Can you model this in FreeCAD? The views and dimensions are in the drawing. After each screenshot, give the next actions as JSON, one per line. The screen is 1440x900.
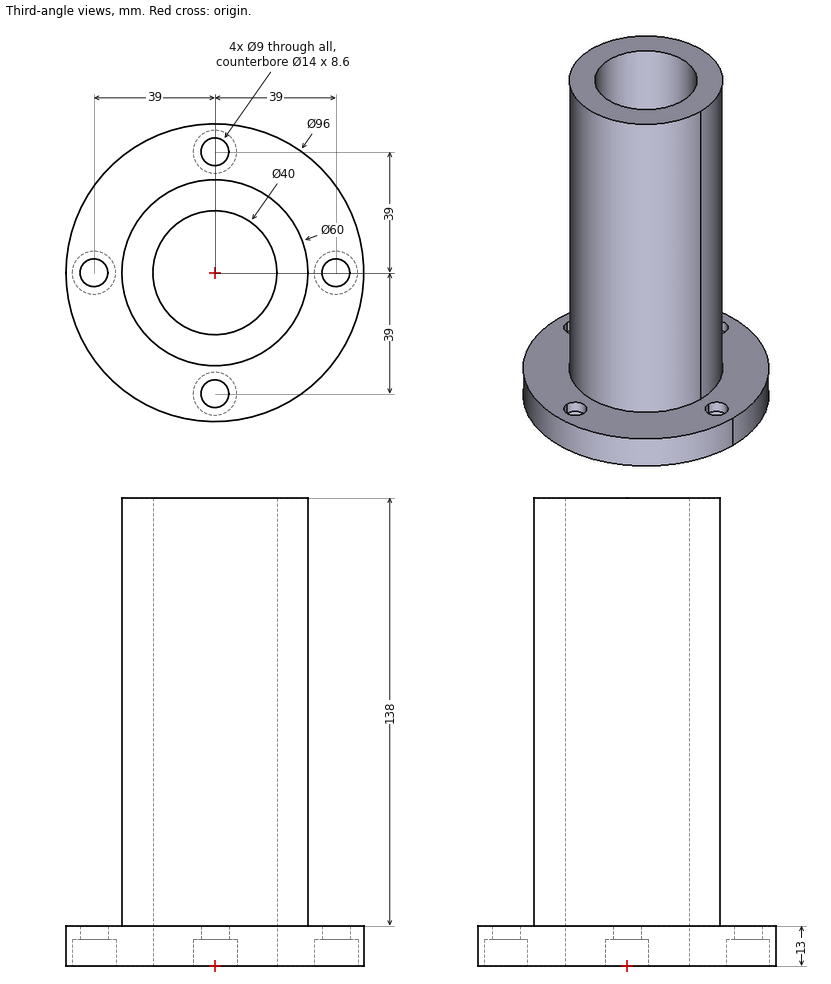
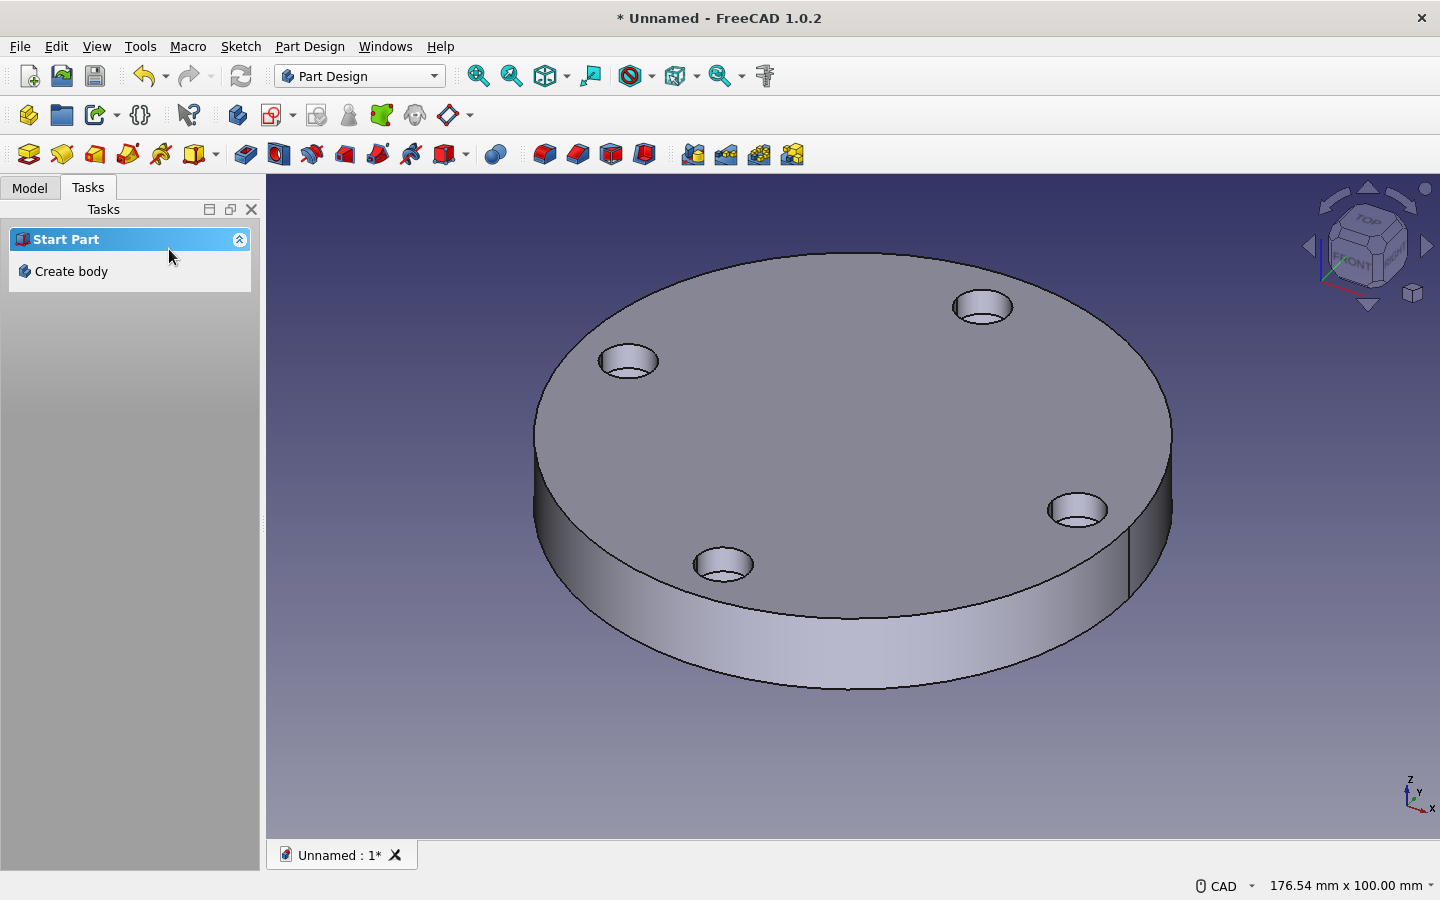
{"action": "left_click", "coordinate": [853, 435]}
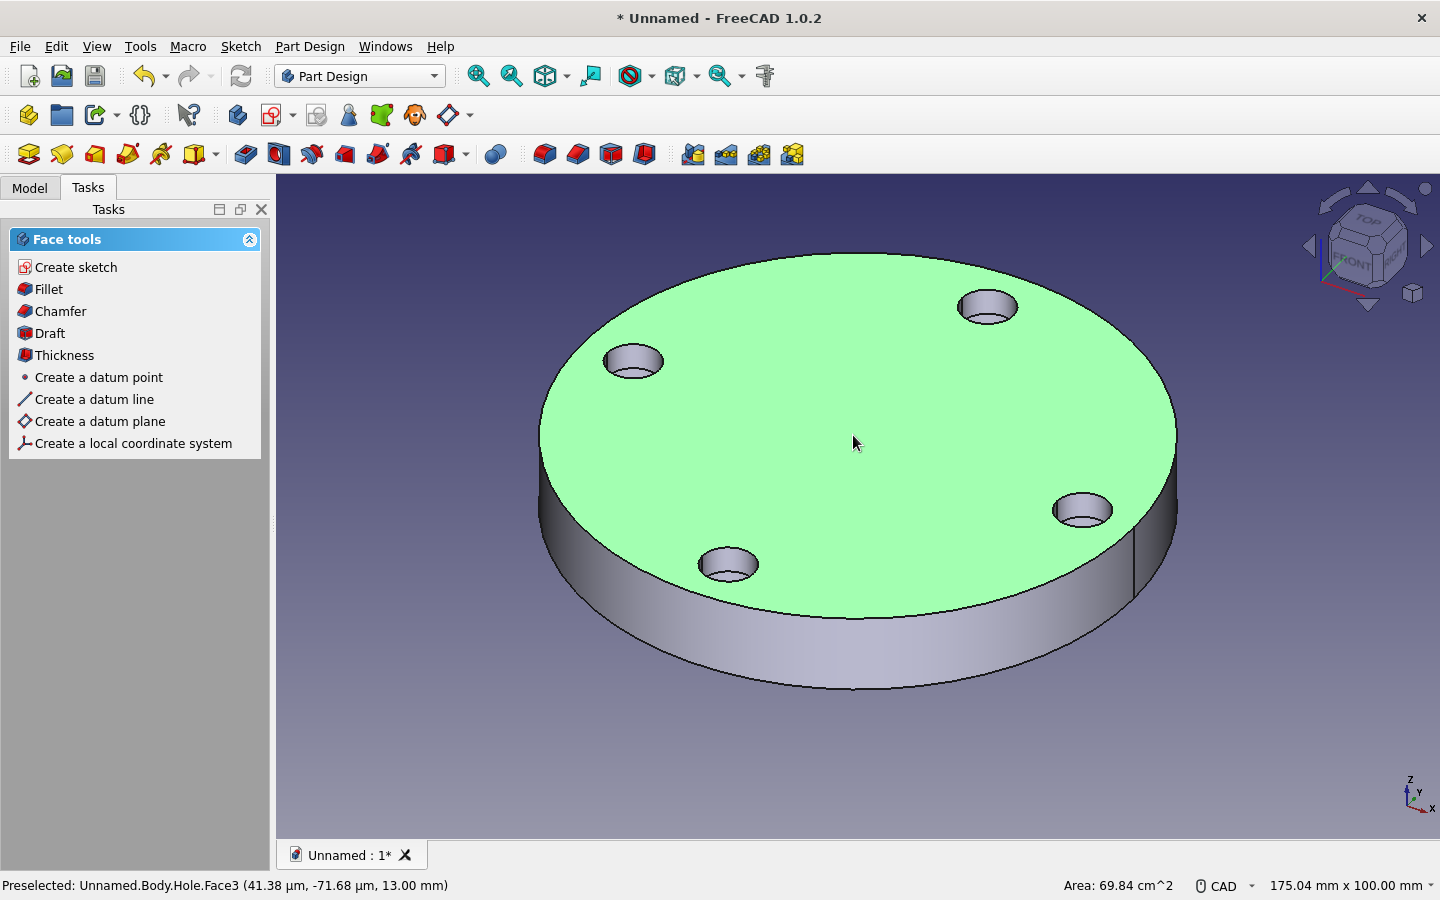
{"action": "left_click", "coordinate": [270, 116]}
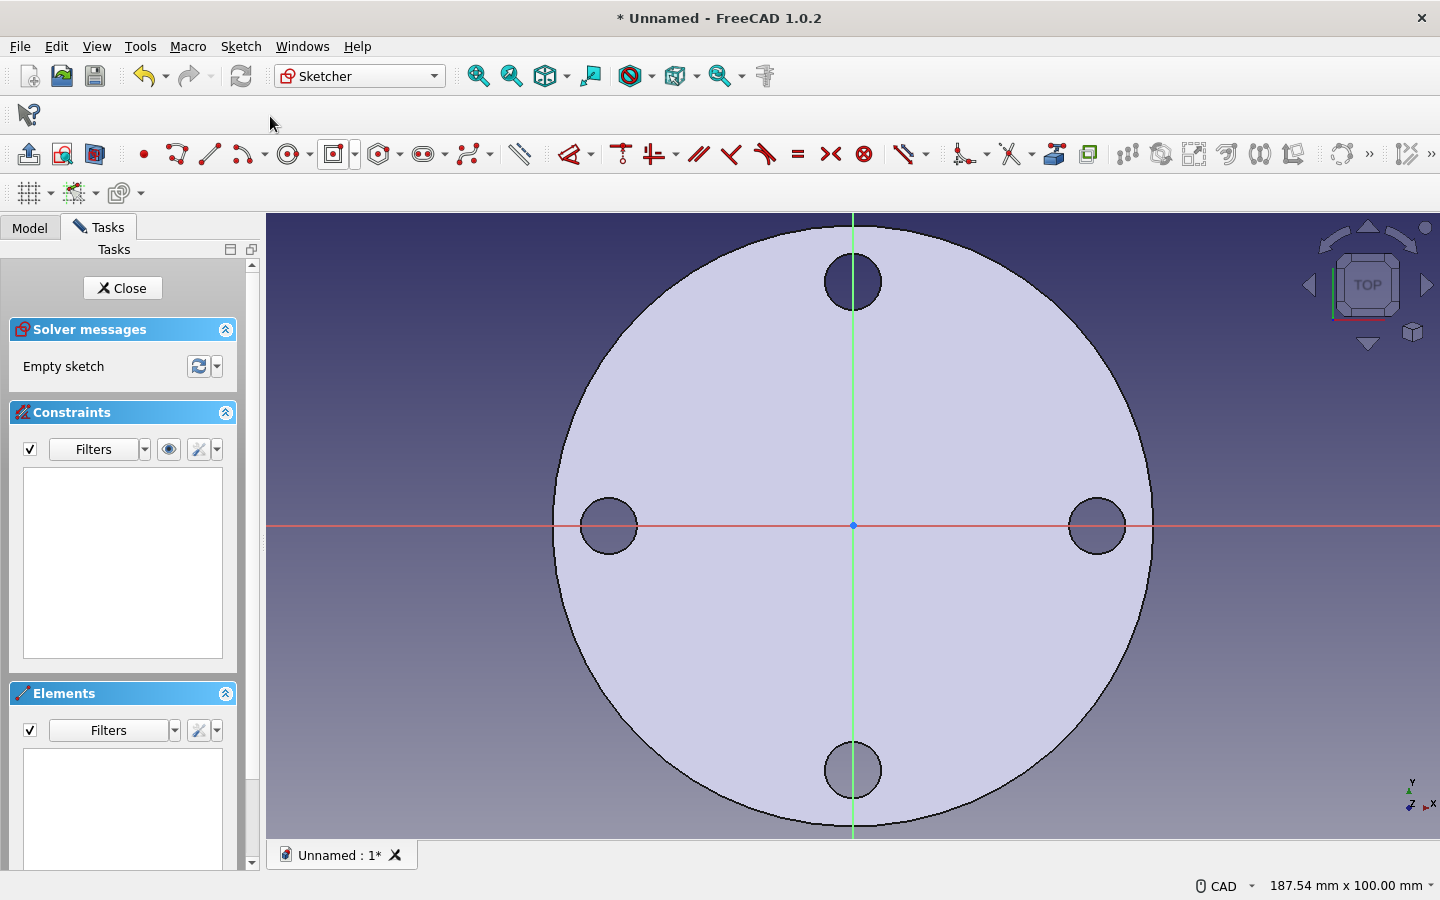
{"action": "left_click", "coordinate": [288, 154]}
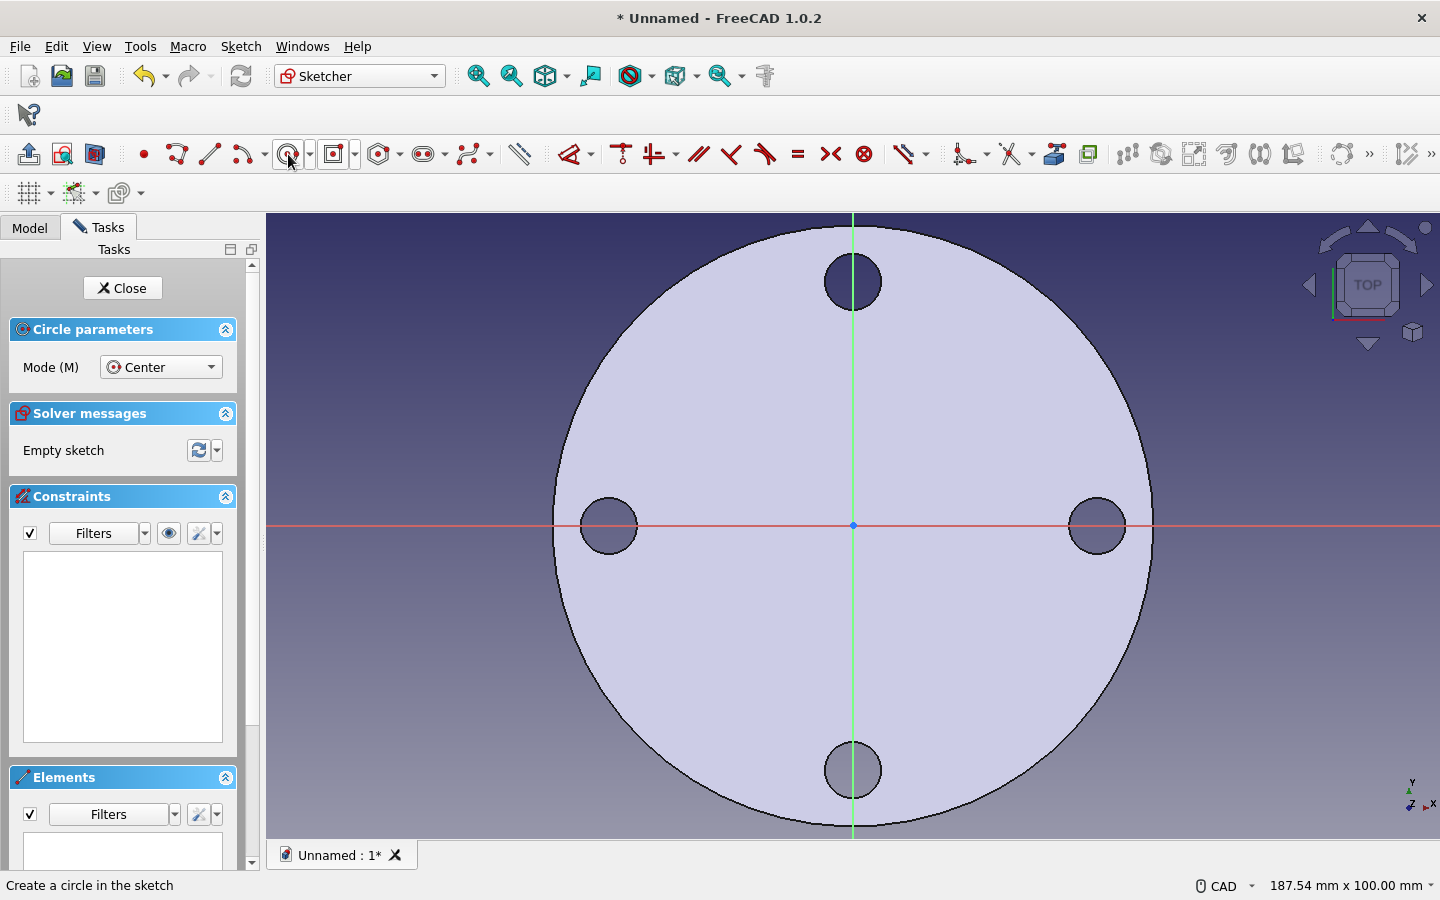
{"action": "left_click", "coordinate": [853, 526]}
{"action": "mouse_move", "coordinate": [986, 393]}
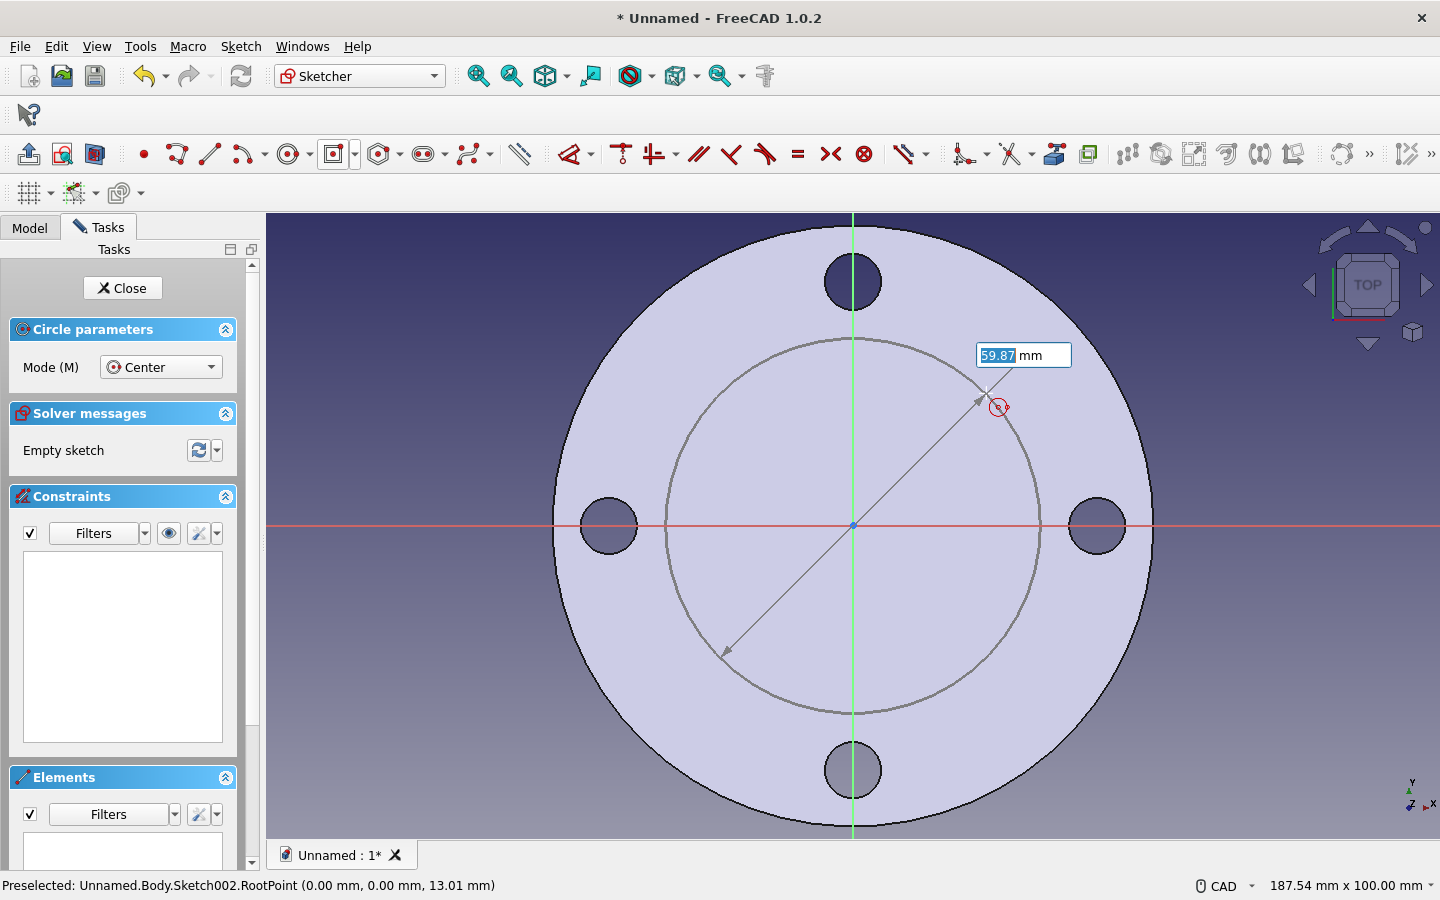
{"action": "type", "text": "60"}
{"action": "key", "text": "Return"}
{"action": "key", "text": "Escape"}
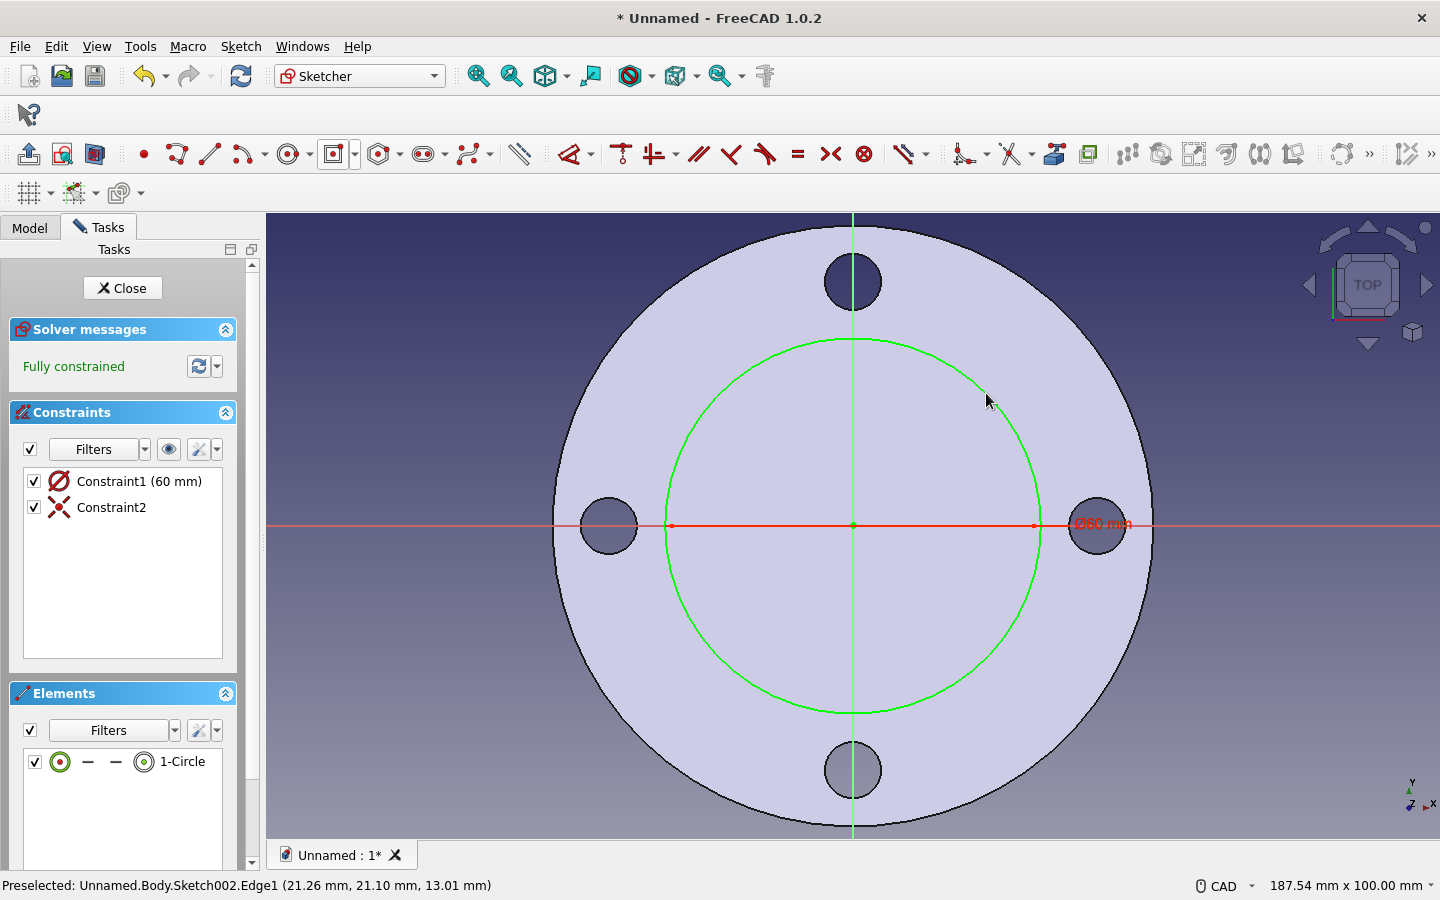
{"action": "left_click", "coordinate": [123, 288]}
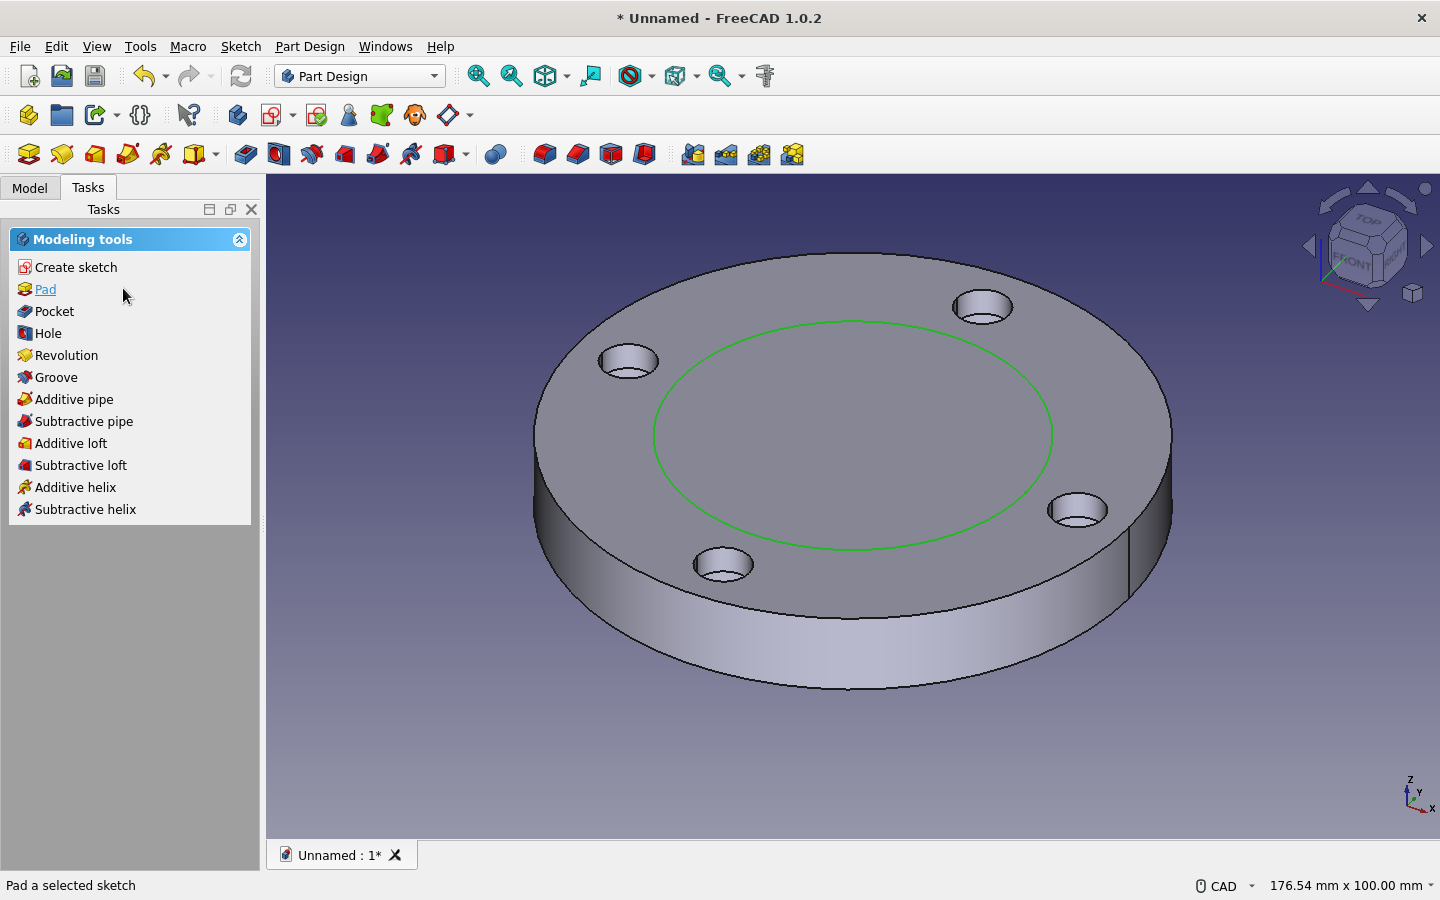
{"action": "left_click", "coordinate": [29, 154]}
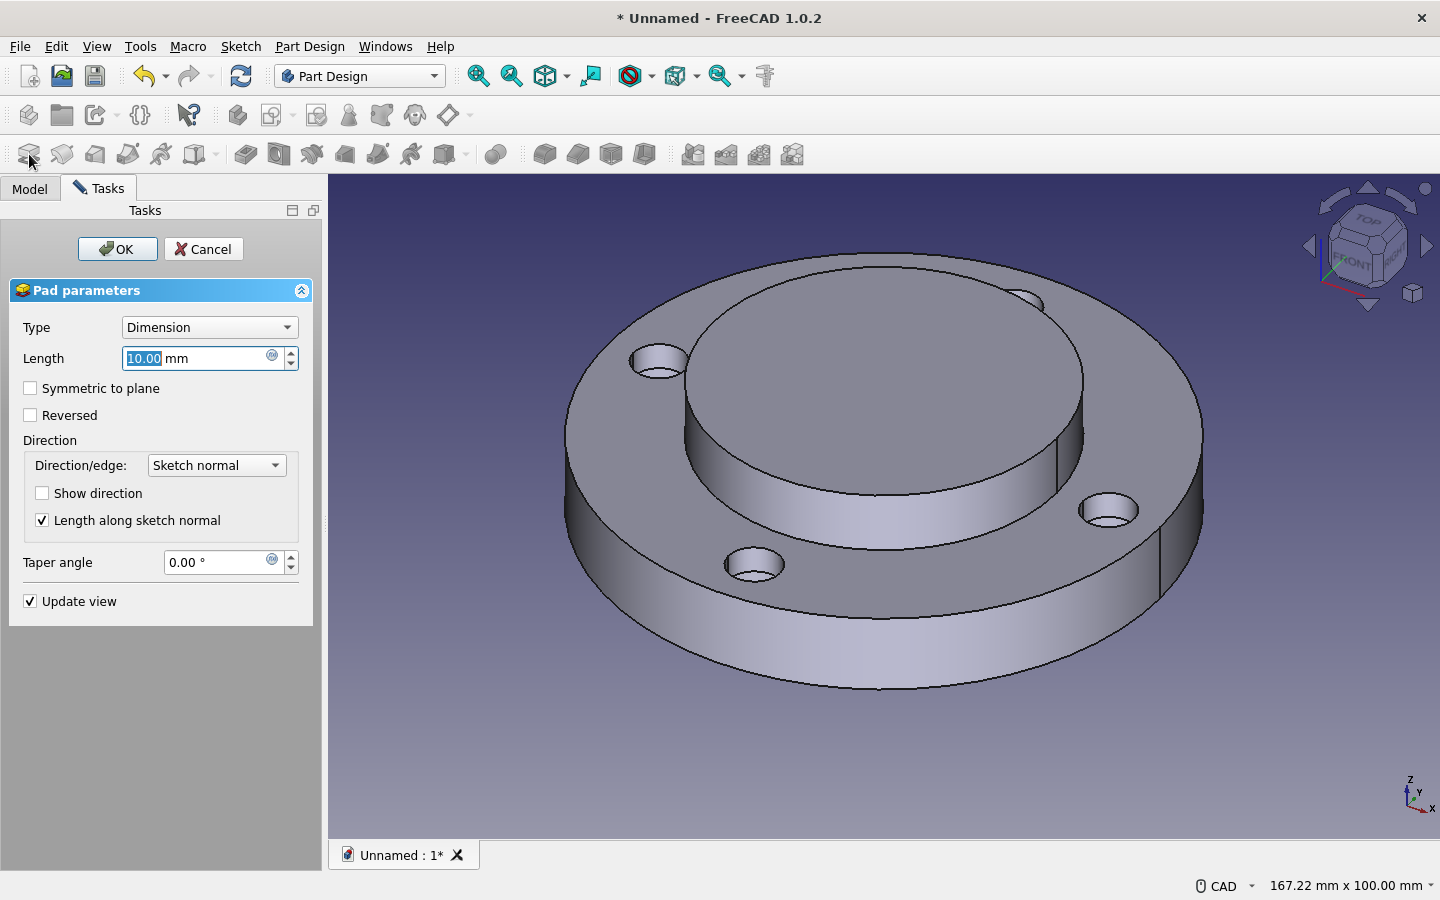
{"action": "type", "text": "138"}
{"action": "key", "text": "Tab"}